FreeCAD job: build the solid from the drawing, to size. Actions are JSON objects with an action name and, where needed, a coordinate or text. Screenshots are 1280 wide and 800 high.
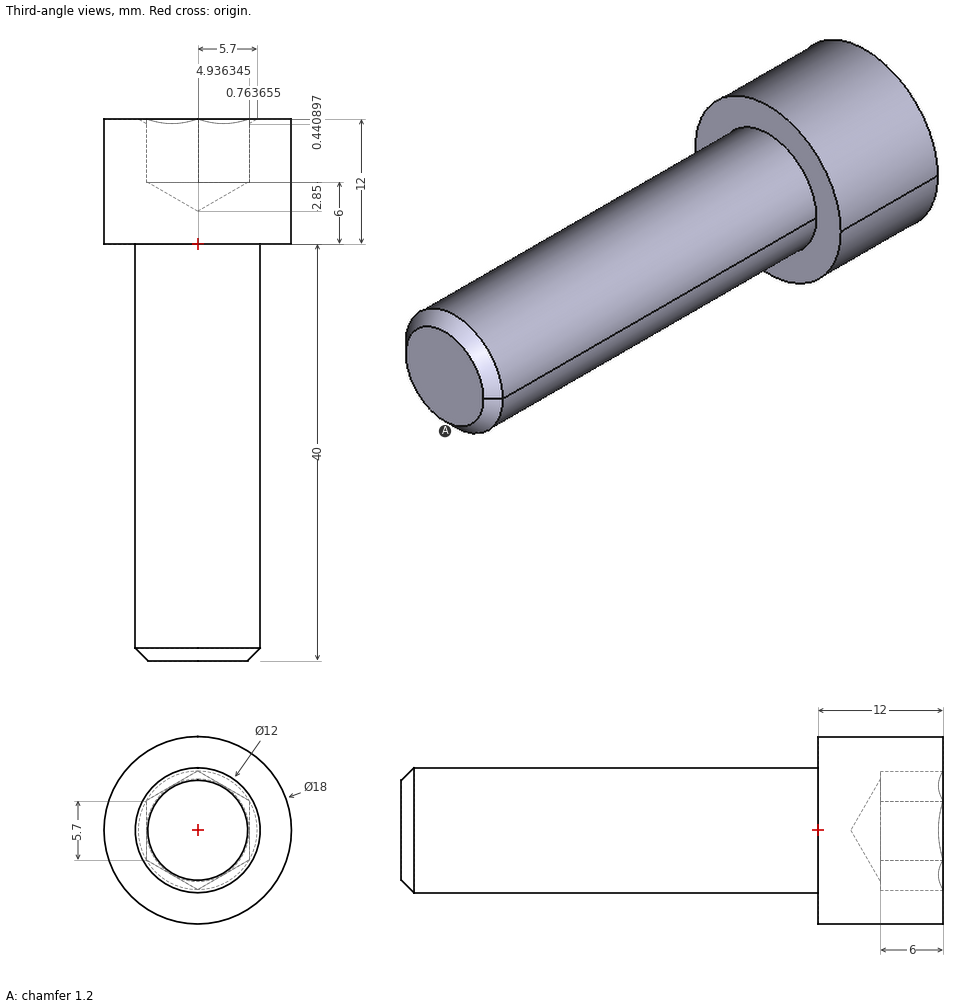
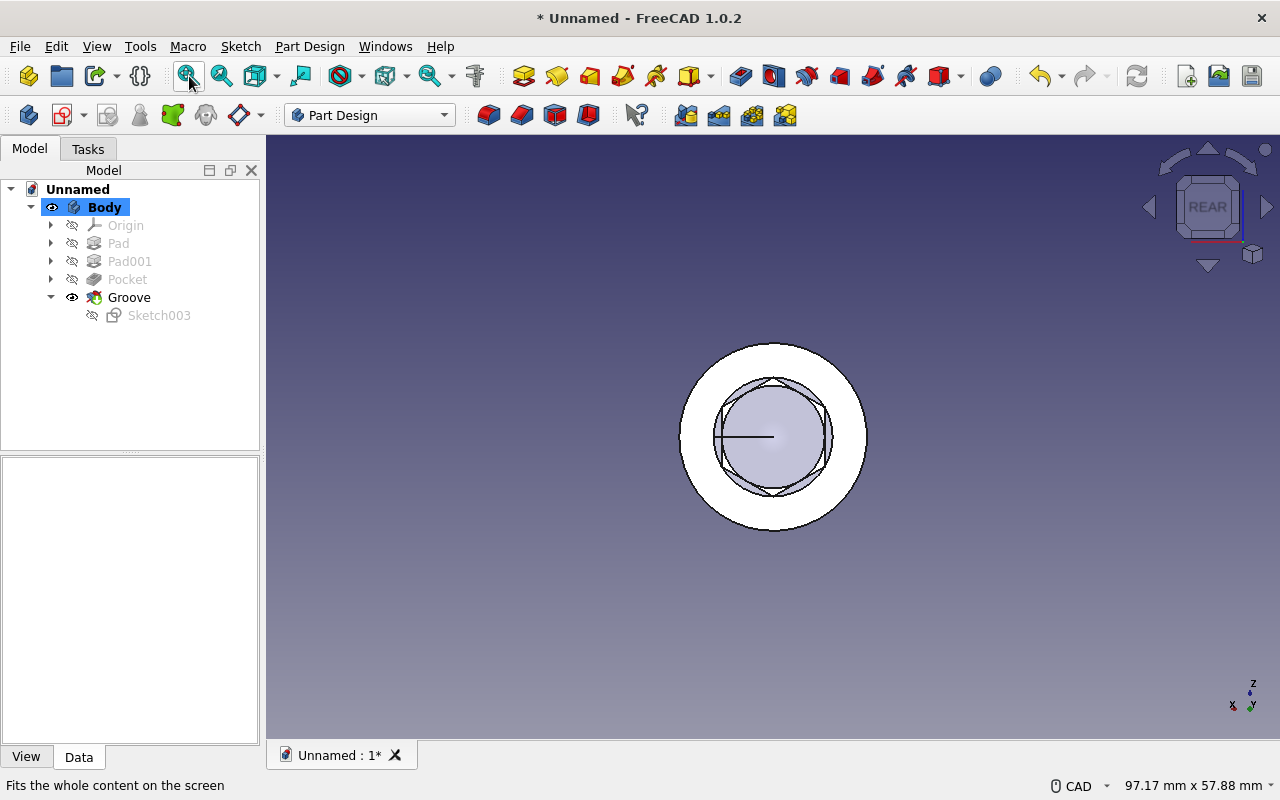
{"action": "key", "text": "0"}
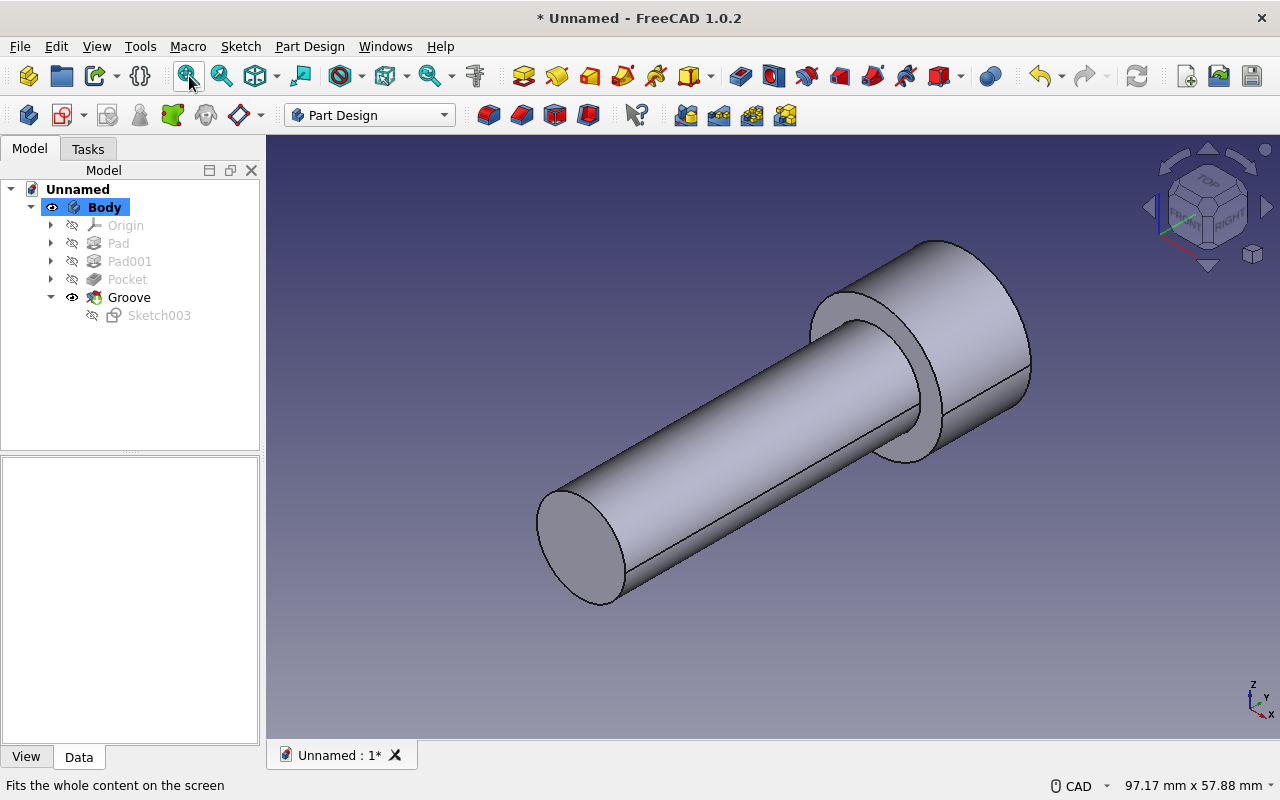
{"action": "left_click", "coordinate": [567, 490]}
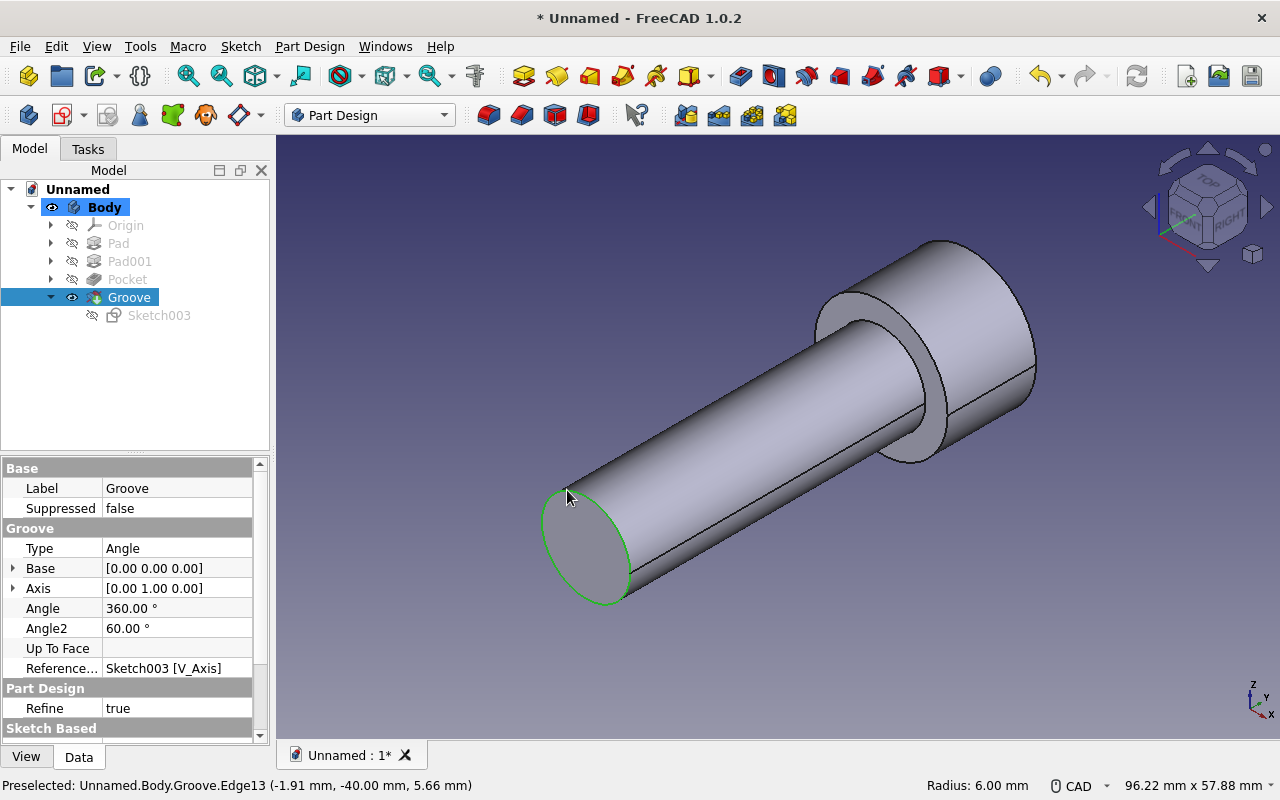
{"action": "left_click", "coordinate": [522, 116]}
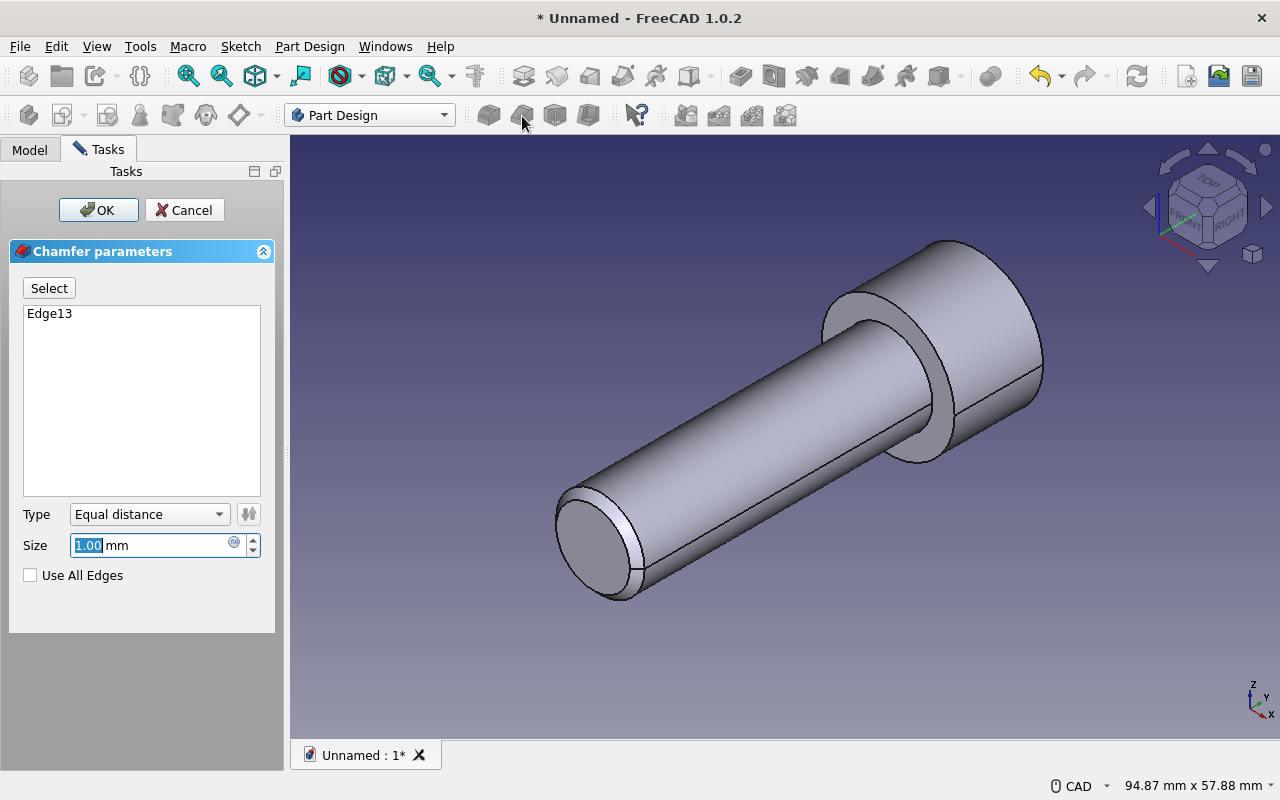
{"action": "type", "text": "1.2"}
{"action": "key", "text": "Tab"}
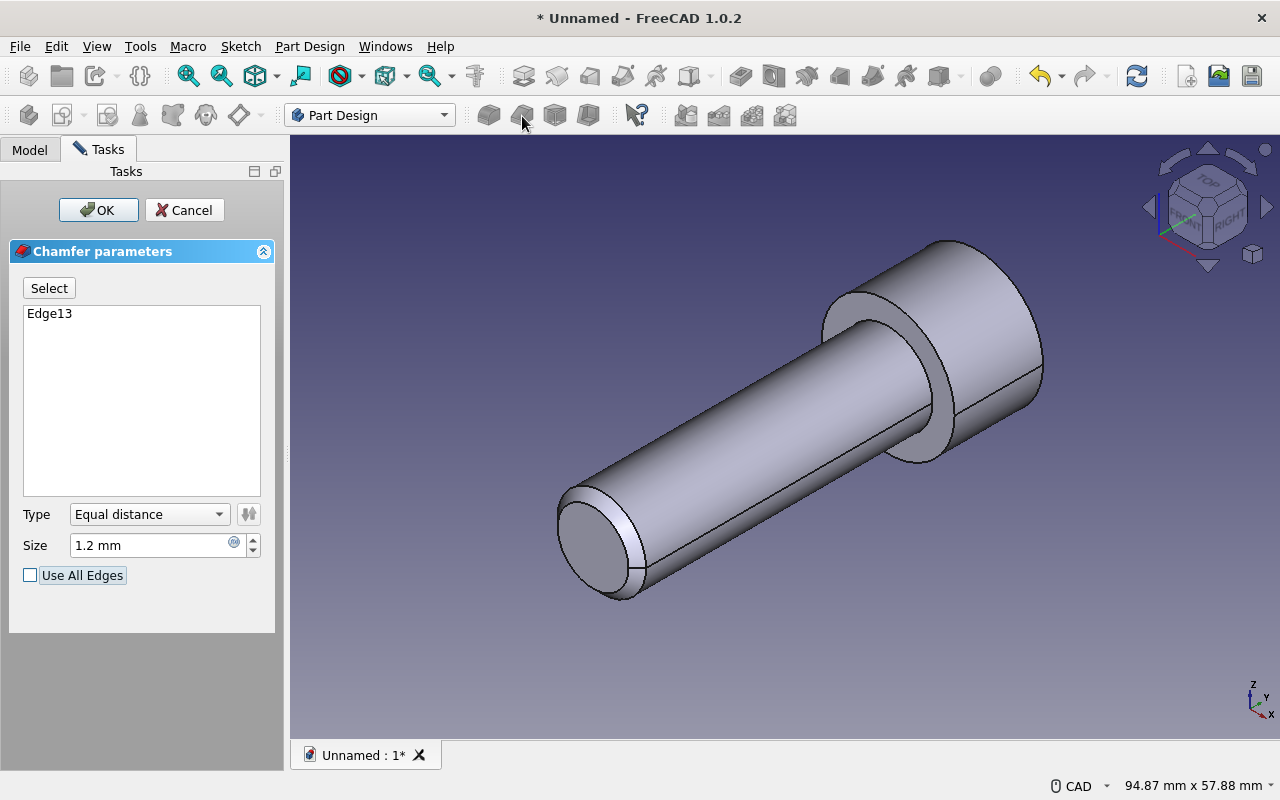
{"action": "left_click", "coordinate": [99, 210]}